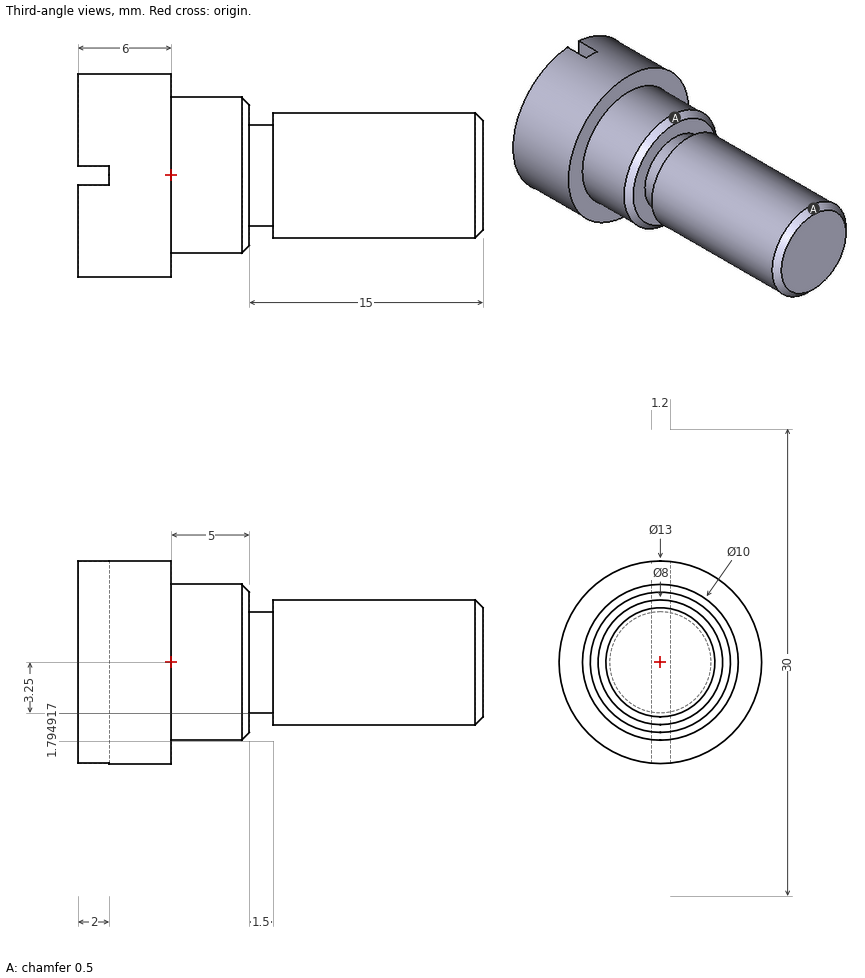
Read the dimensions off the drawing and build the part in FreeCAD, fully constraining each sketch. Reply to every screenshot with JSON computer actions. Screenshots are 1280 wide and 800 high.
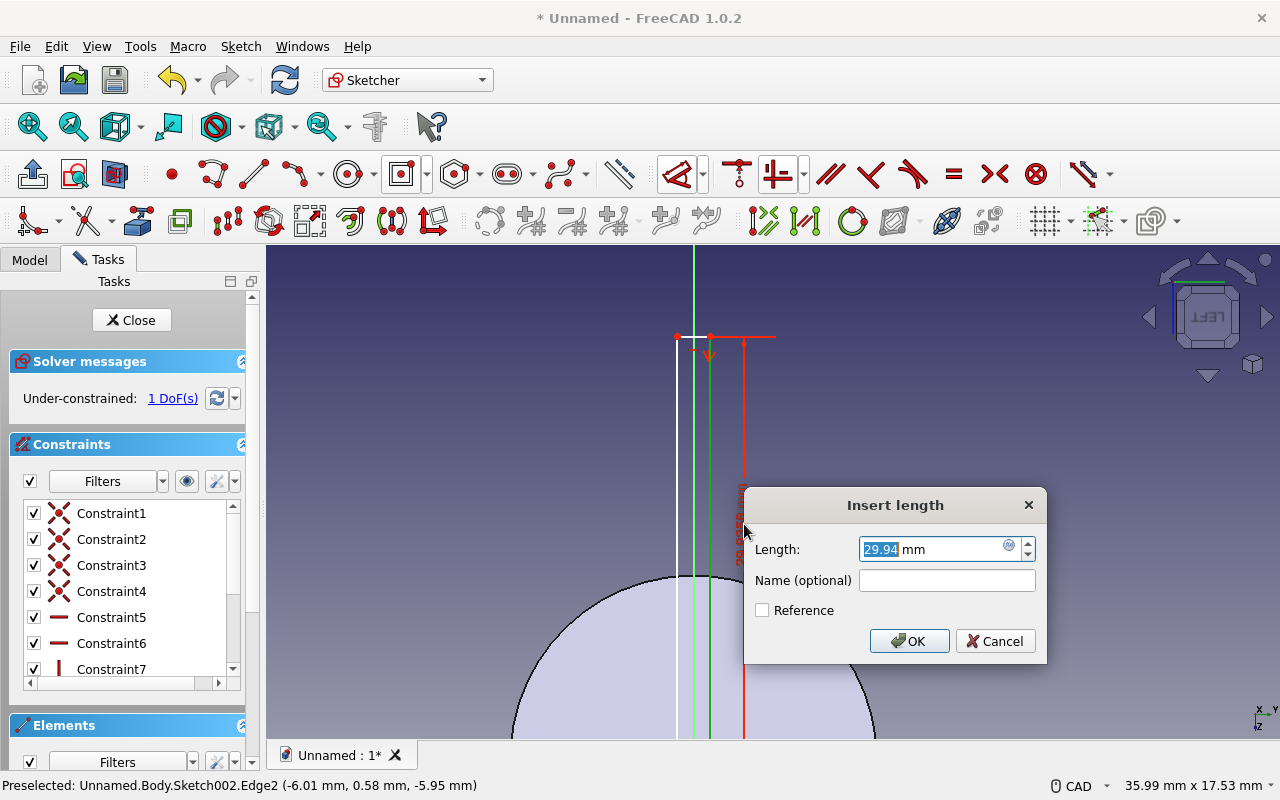
{"action": "type", "text": "30"}
{"action": "key", "text": "Return"}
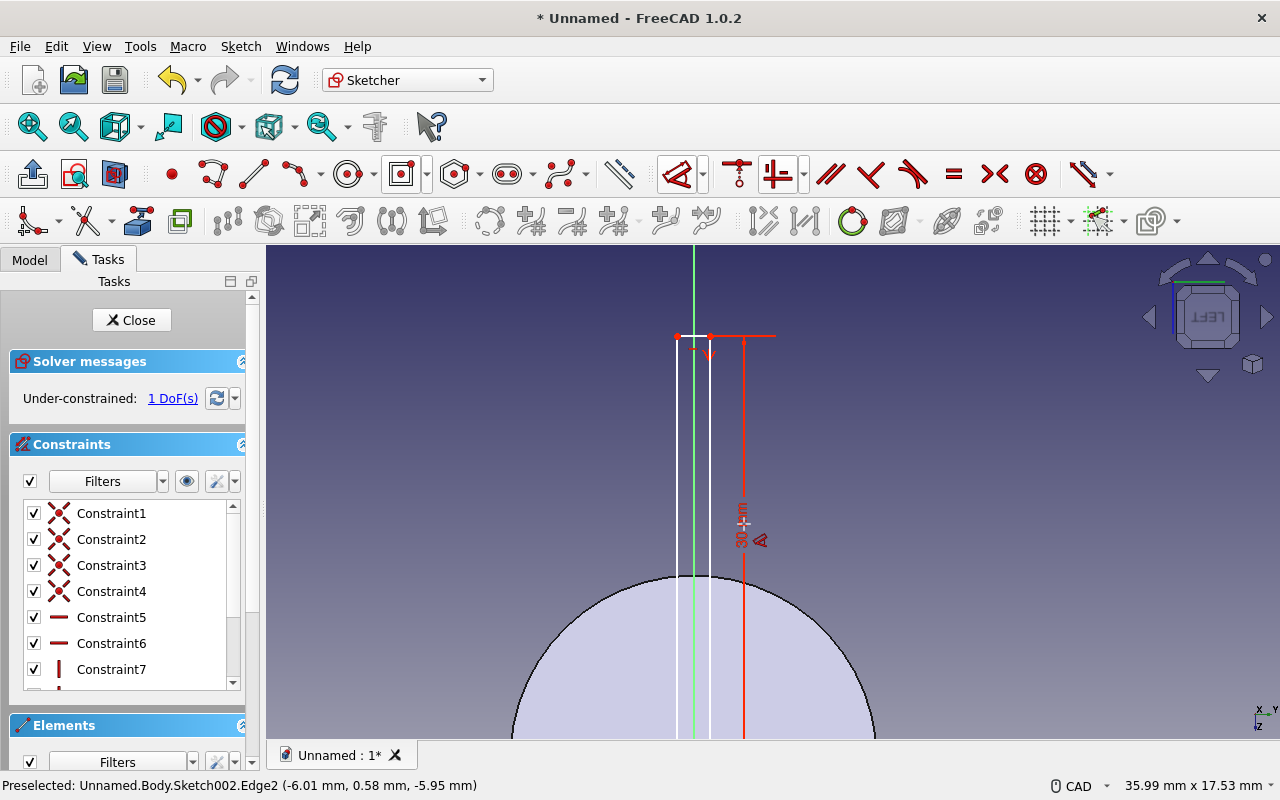
{"action": "scroll", "coordinate": [711, 337], "scroll_direction": "down", "scroll_amount": 5}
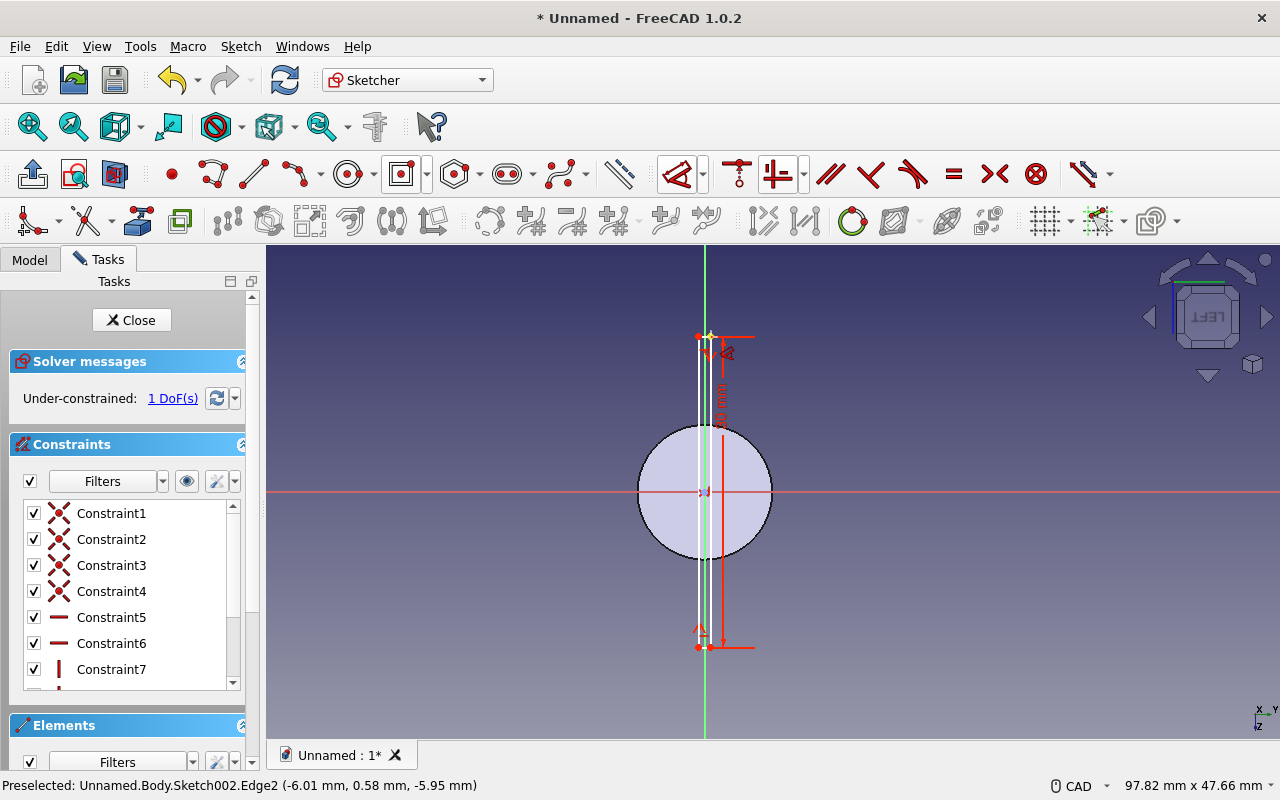
{"action": "scroll", "coordinate": [704, 648], "scroll_direction": "up", "scroll_amount": 6}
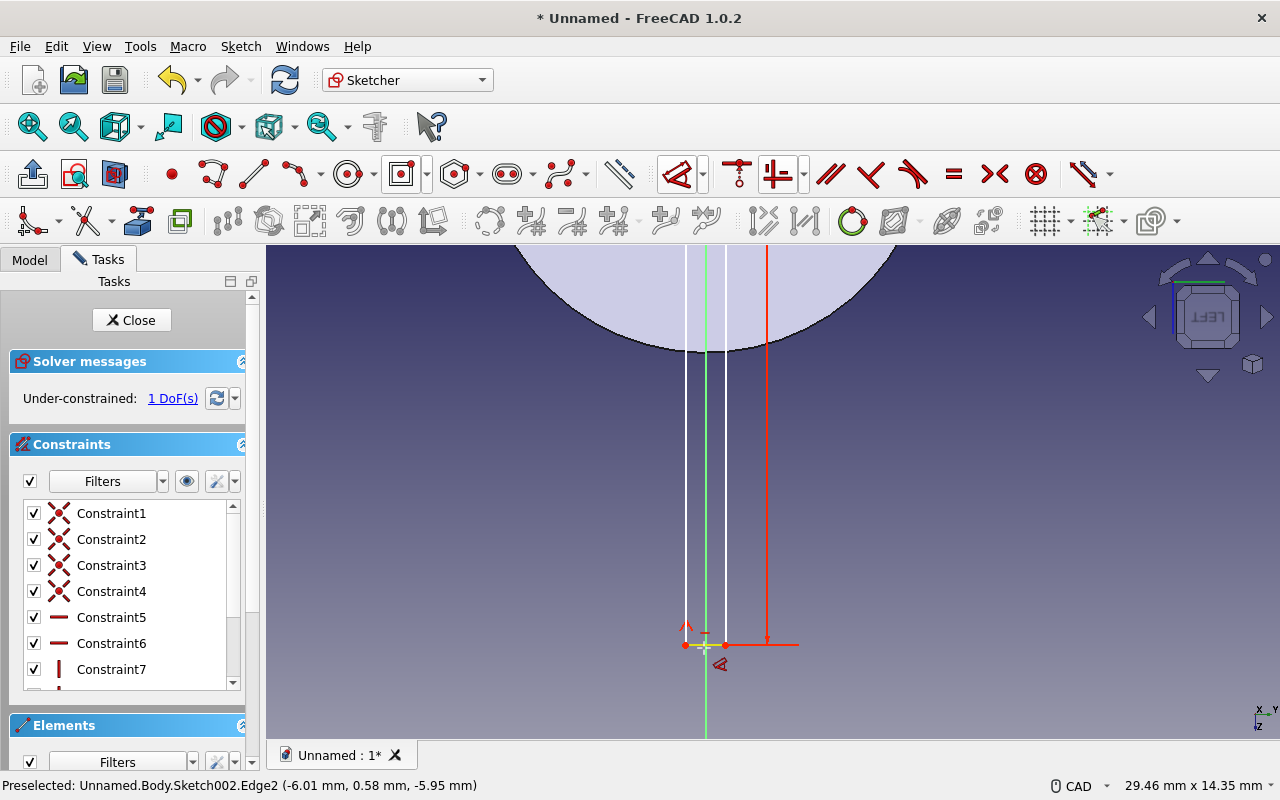
{"action": "left_click", "coordinate": [702, 645]}
{"action": "left_click", "coordinate": [692, 679]}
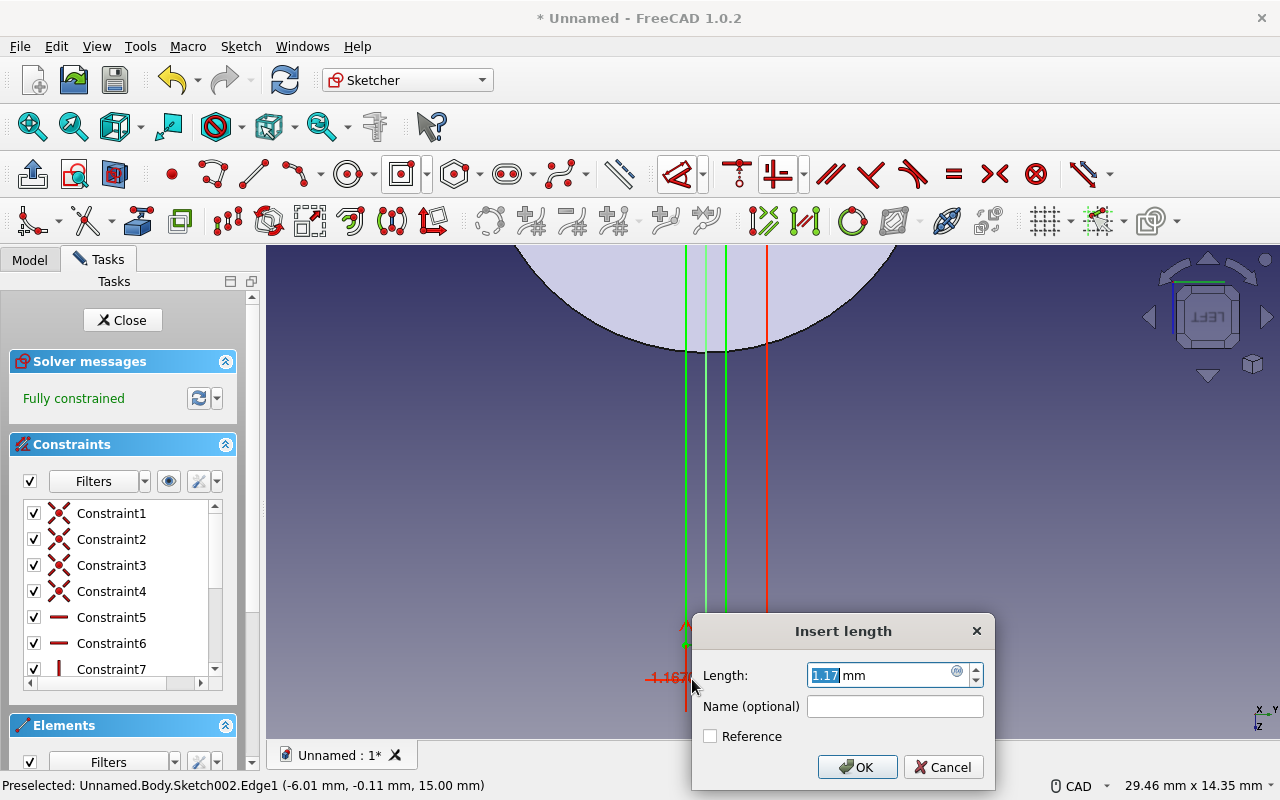
{"action": "type", "text": "1.2"}
{"action": "key", "text": "Return"}
{"action": "key", "text": "Escape"}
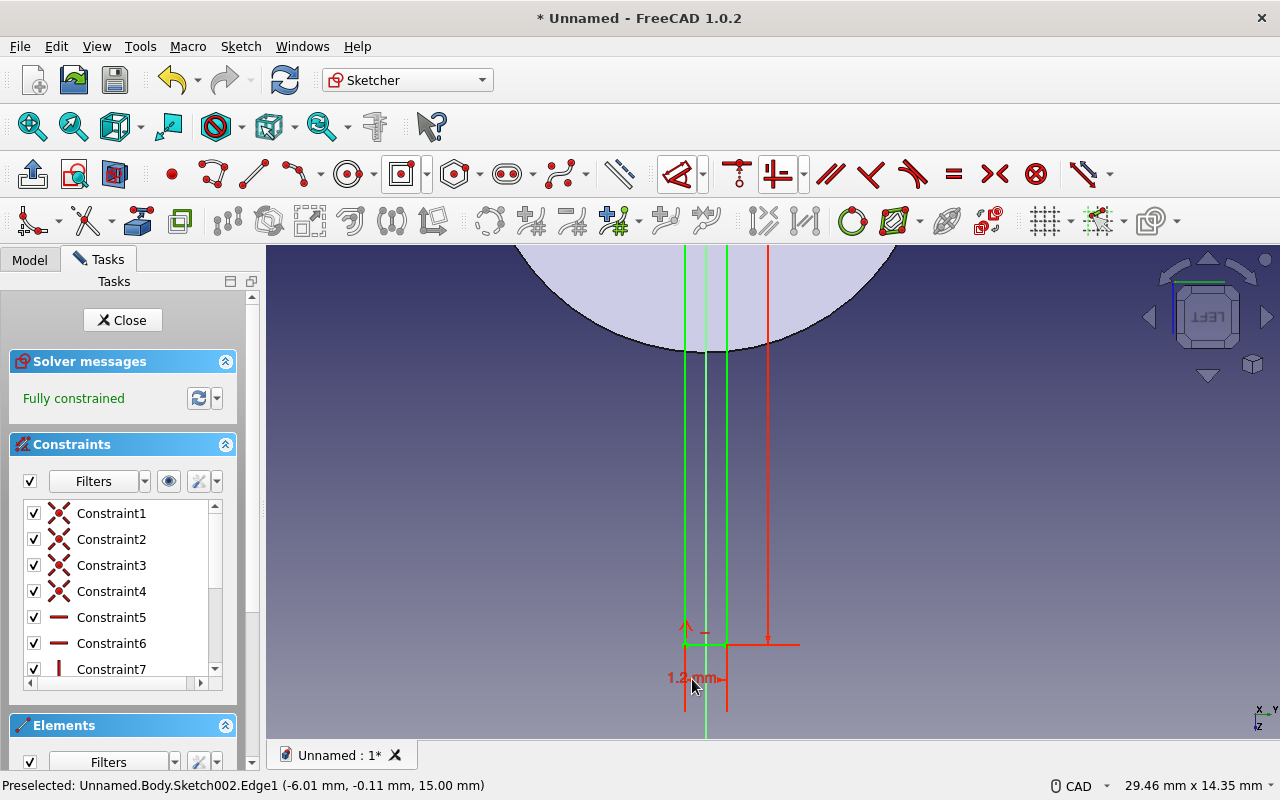
{"action": "left_click", "coordinate": [123, 320]}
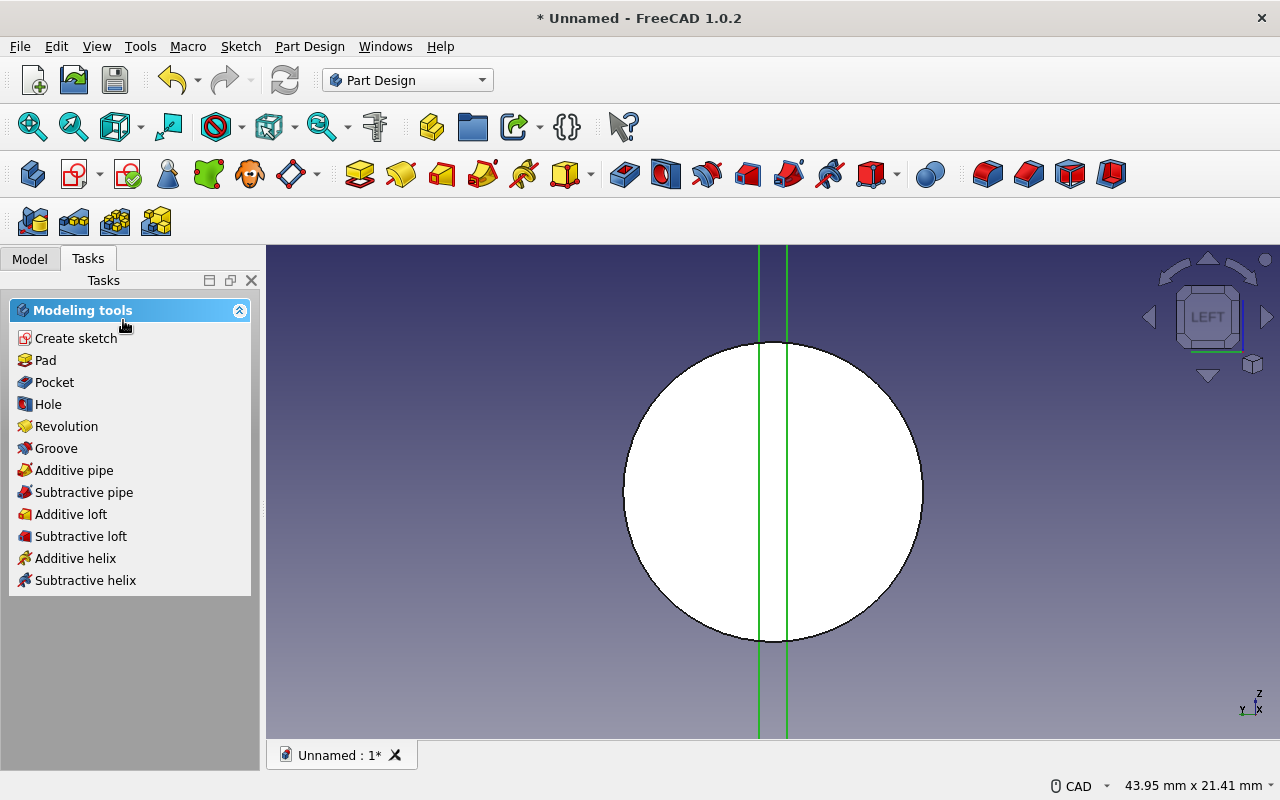
{"action": "left_click", "coordinate": [625, 174]}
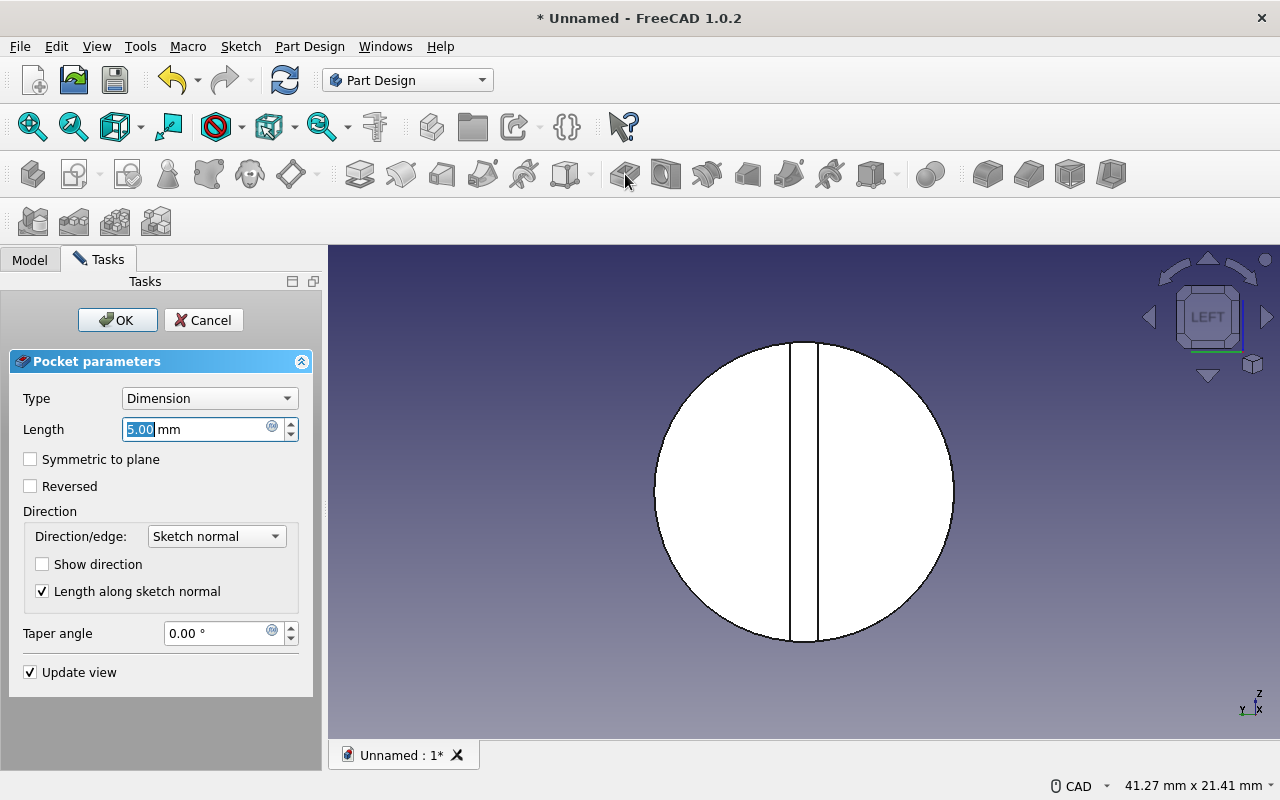
{"action": "type", "text": "2"}
{"action": "key", "text": "Tab"}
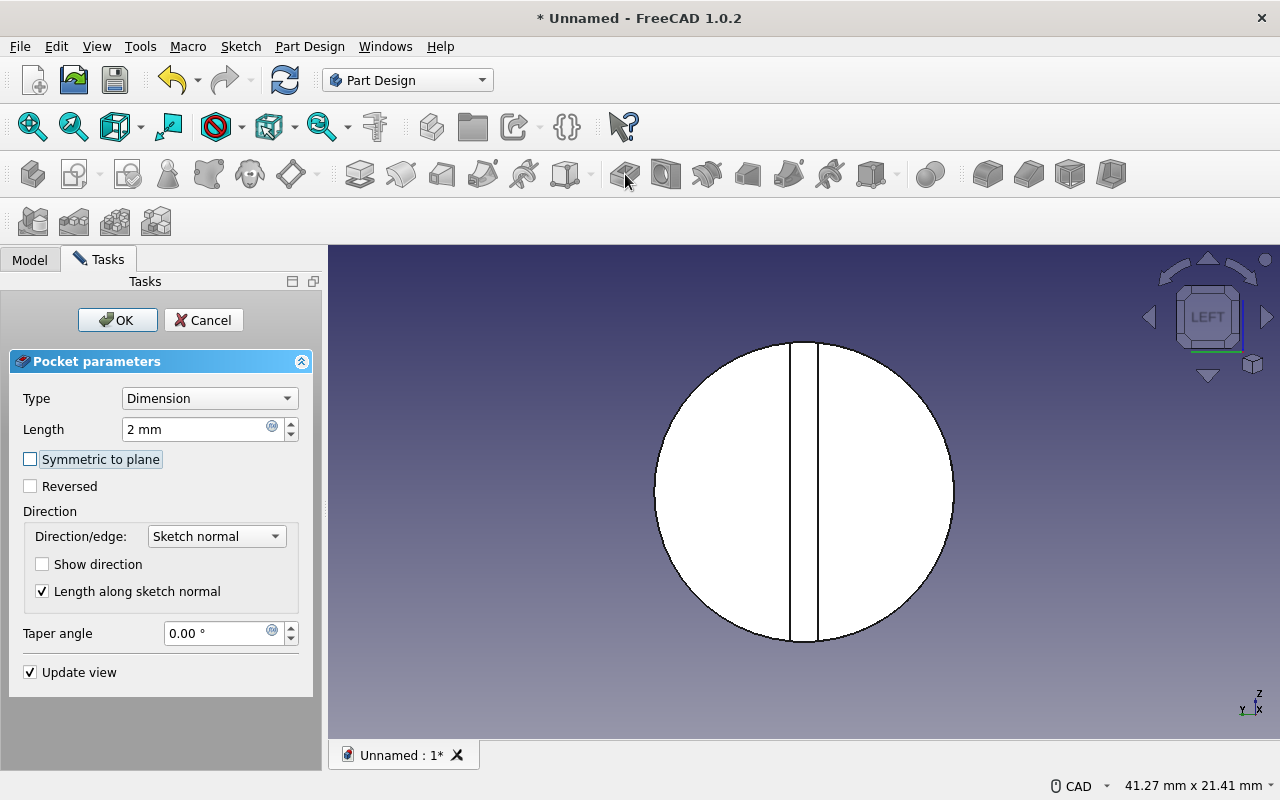
{"action": "left_click", "coordinate": [118, 320]}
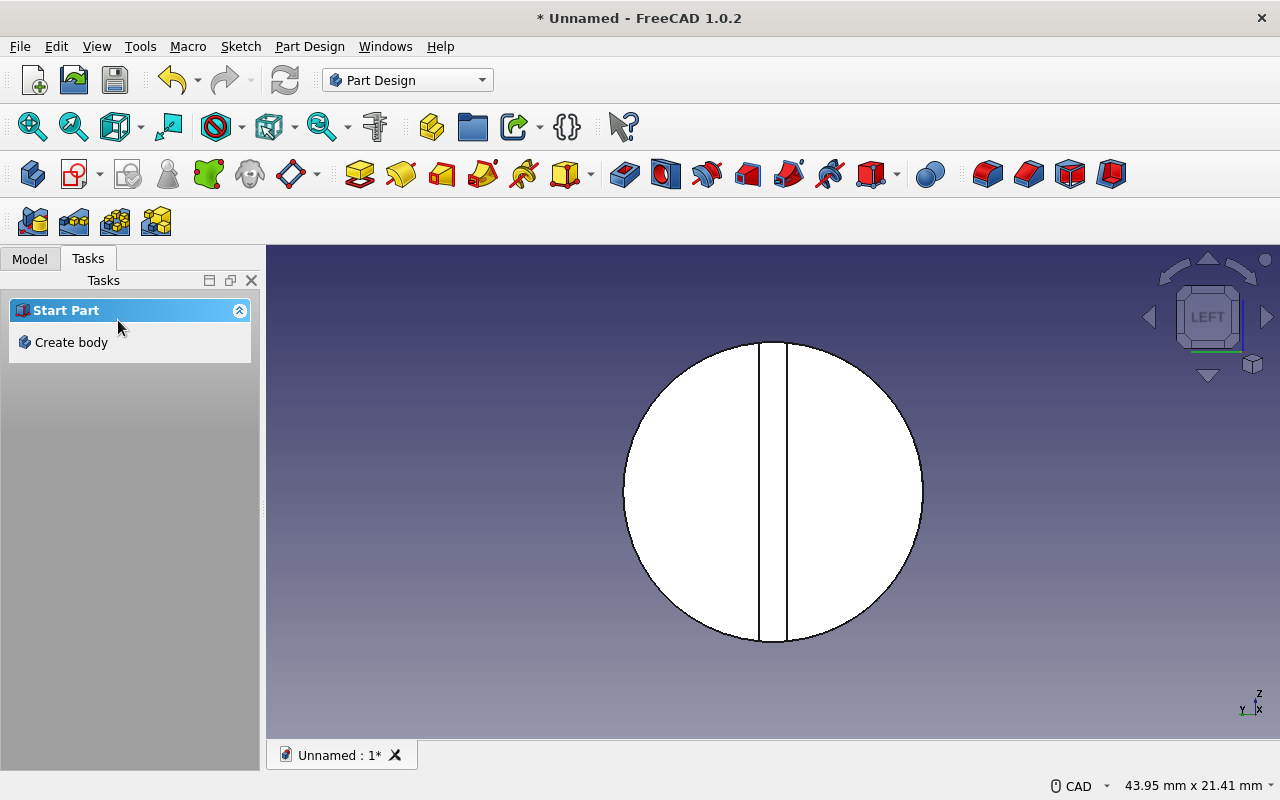
{"action": "key", "text": "0"}